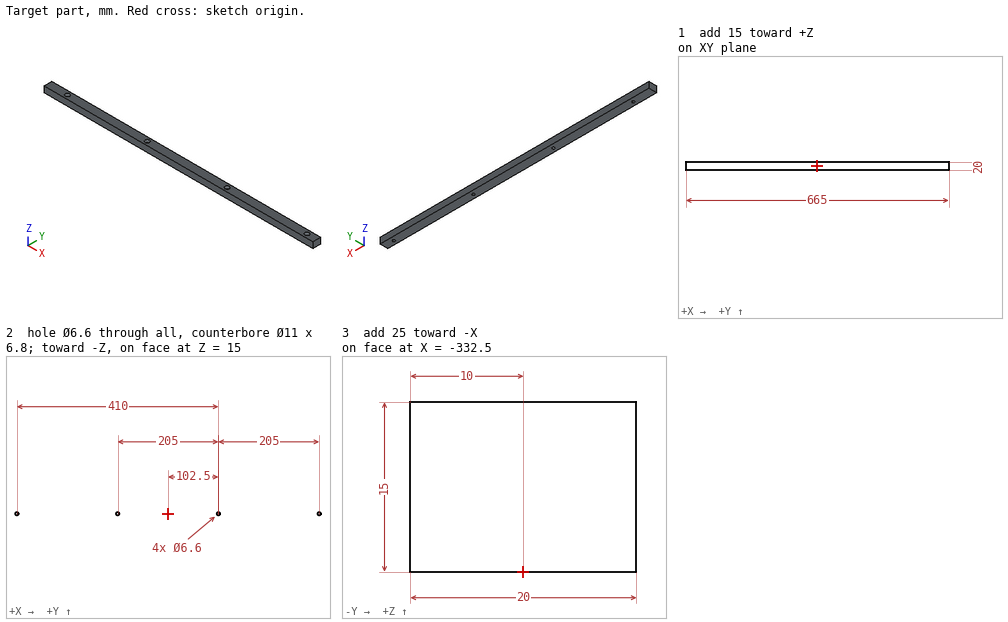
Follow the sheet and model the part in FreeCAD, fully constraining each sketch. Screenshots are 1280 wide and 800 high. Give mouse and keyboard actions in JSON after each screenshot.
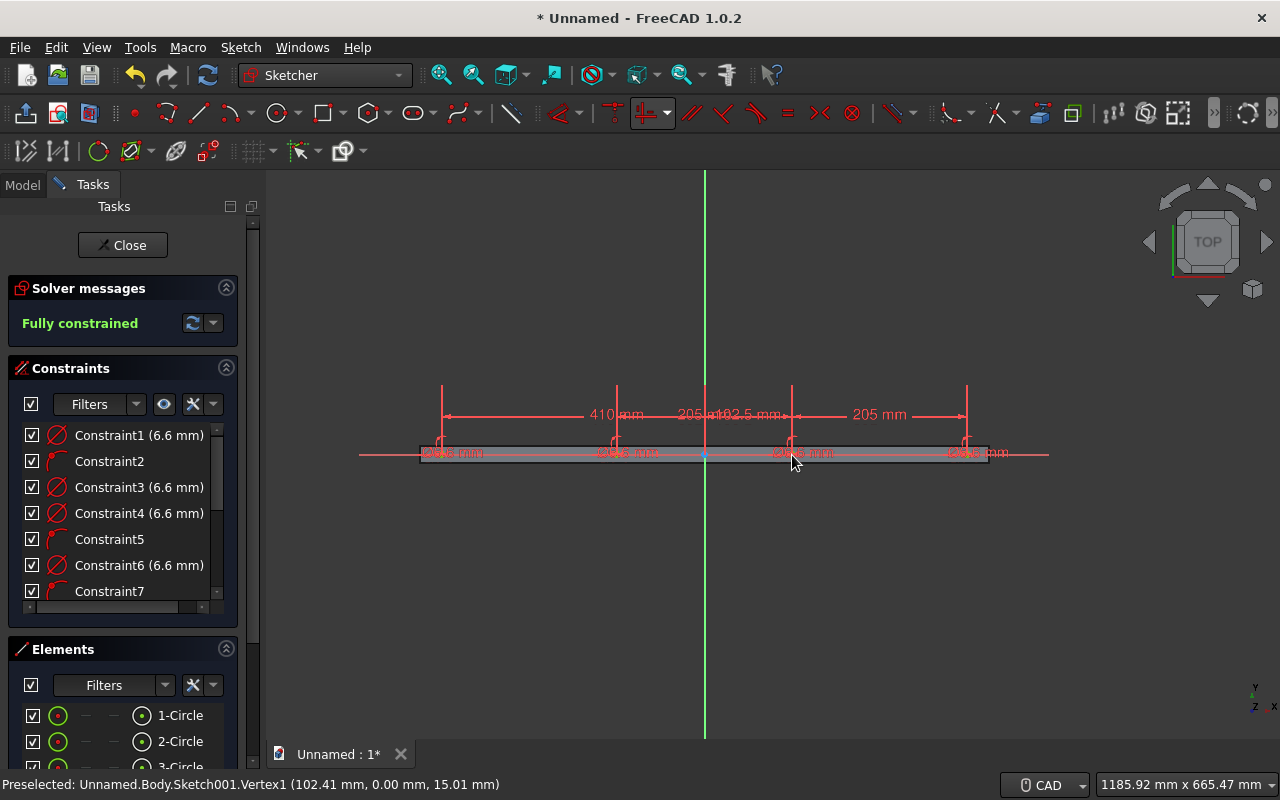
{"action": "left_click", "coordinate": [123, 245]}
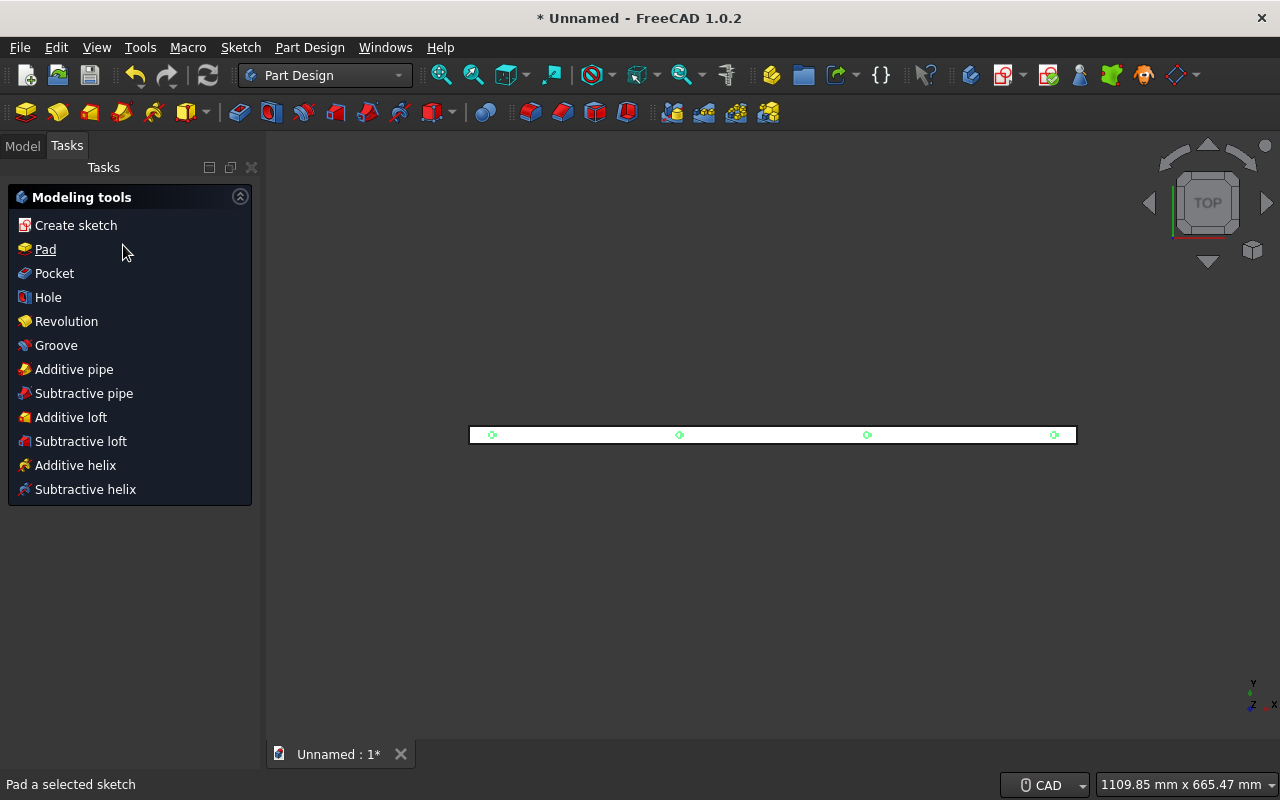
{"action": "left_click", "coordinate": [272, 112]}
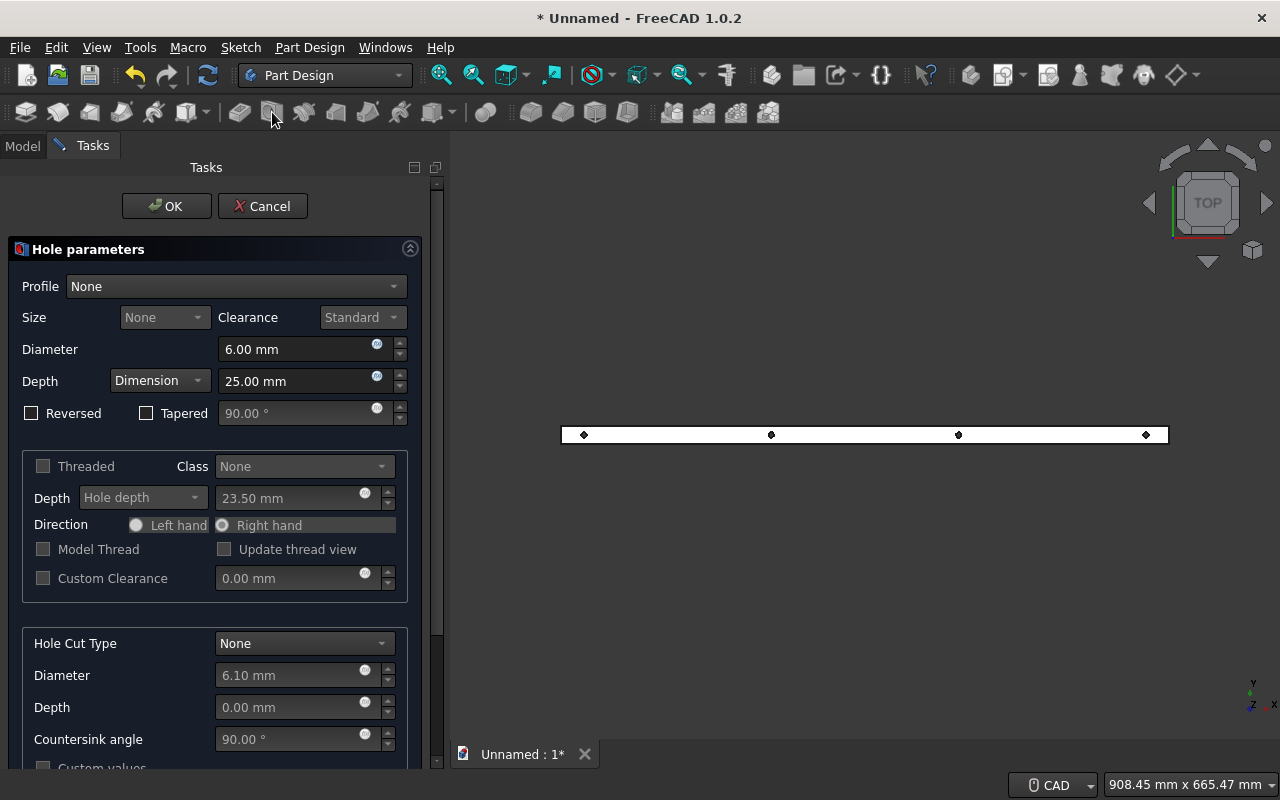
{"action": "triple_click", "coordinate": [305, 349]}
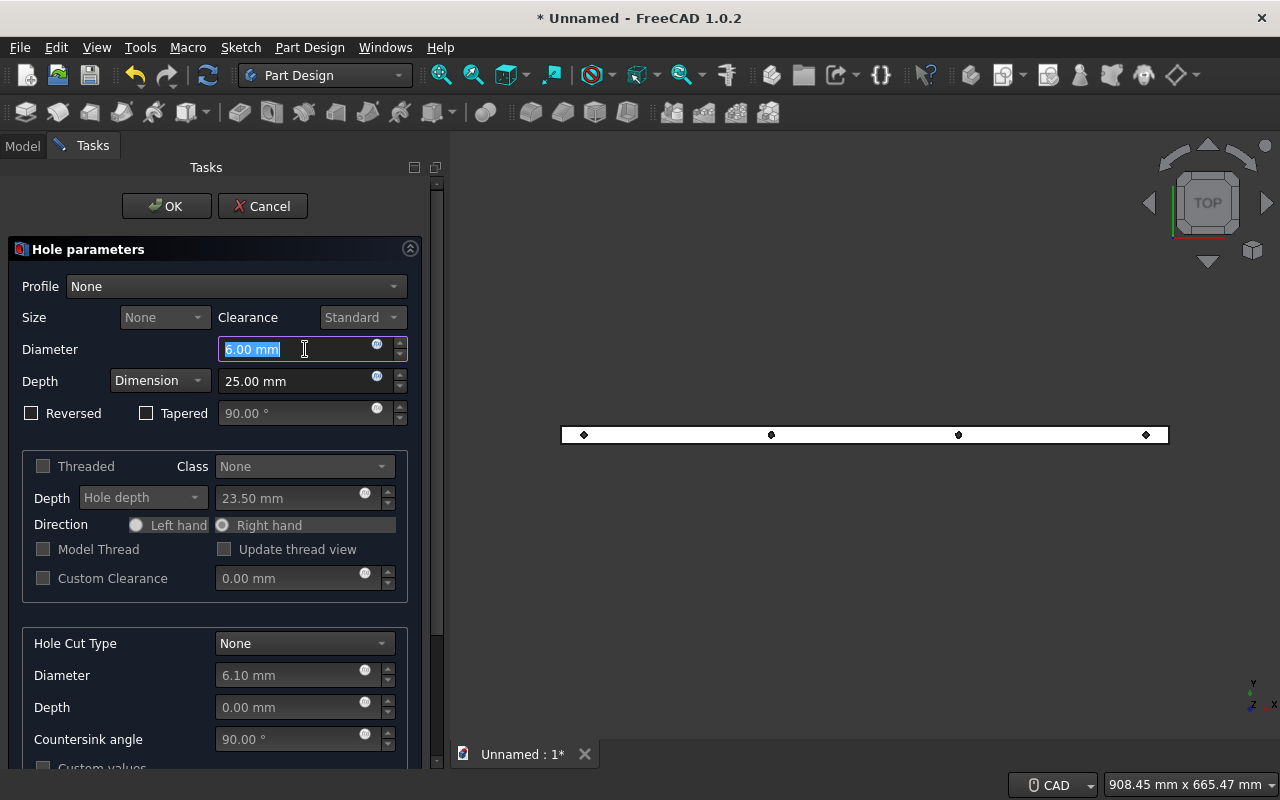
{"action": "type", "text": "6.6"}
{"action": "key", "text": "Tab"}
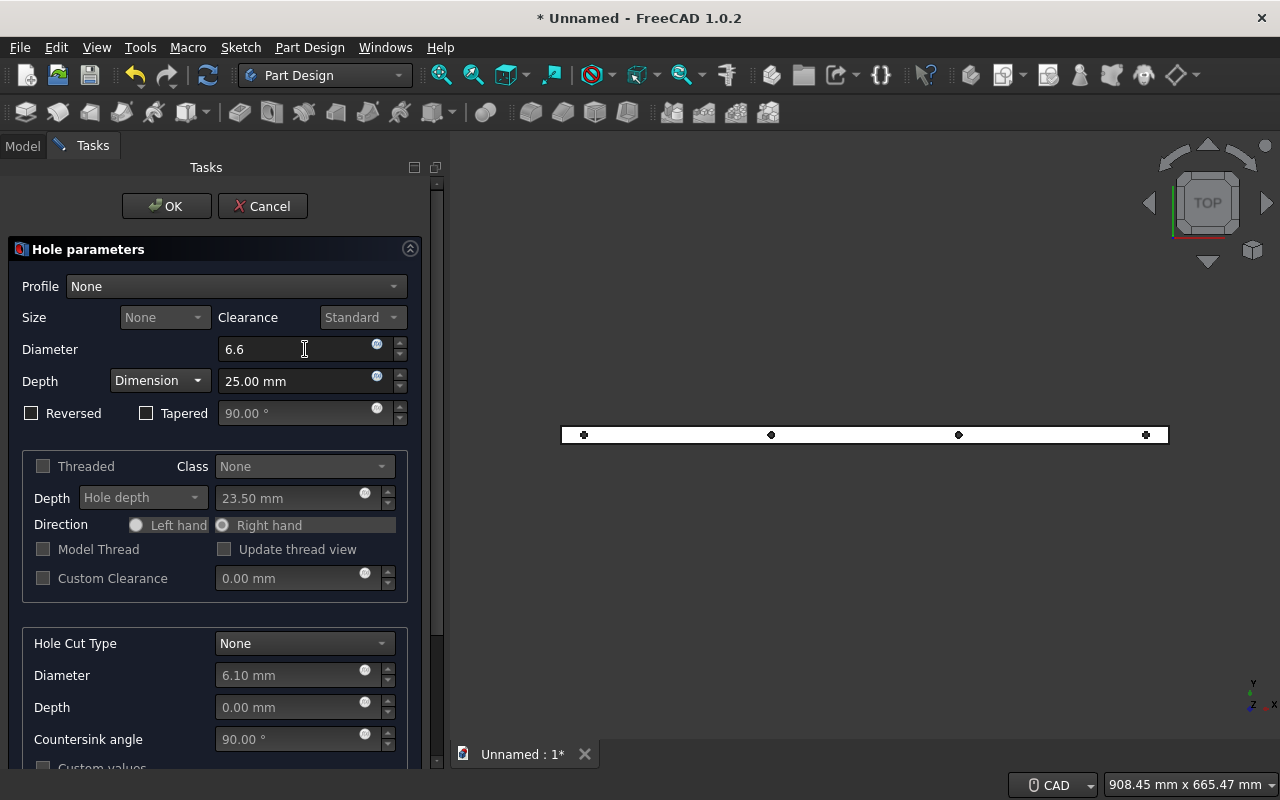
{"action": "left_click", "coordinate": [161, 380]}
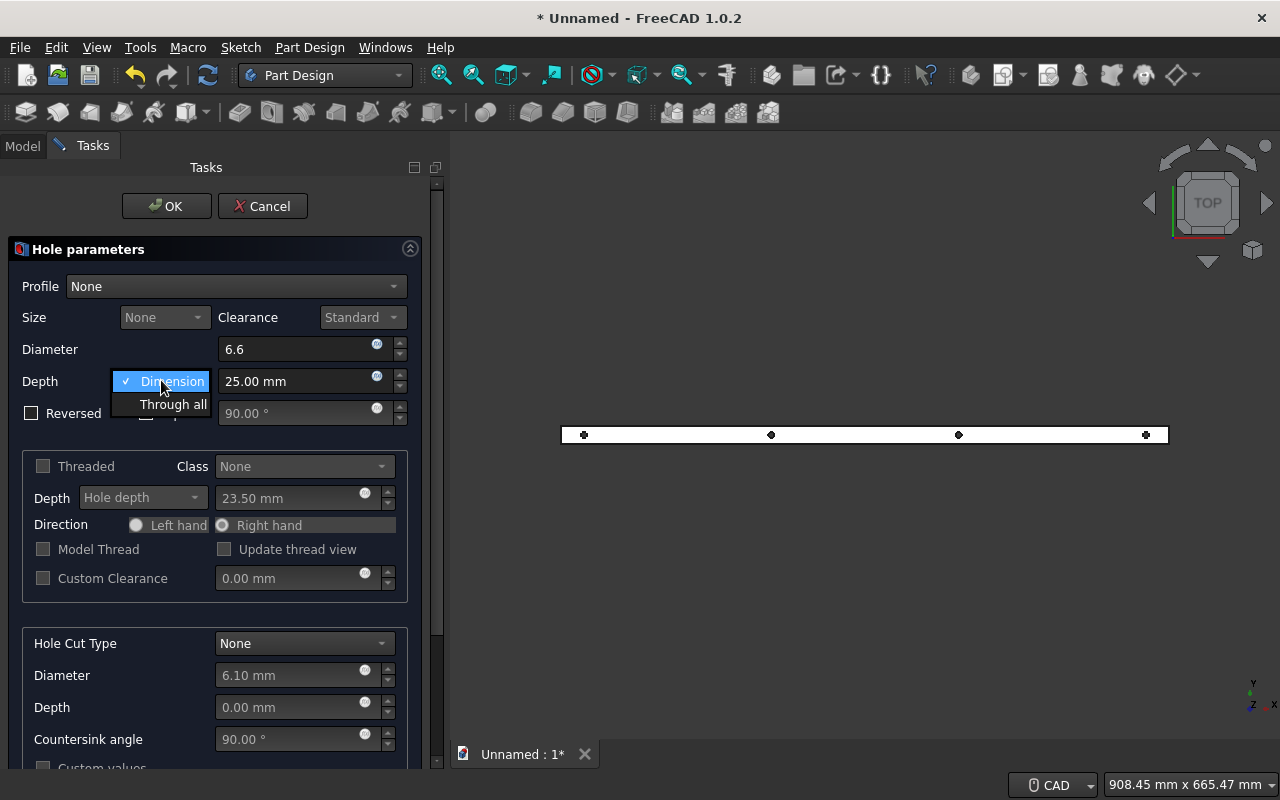
{"action": "left_click", "coordinate": [160, 404]}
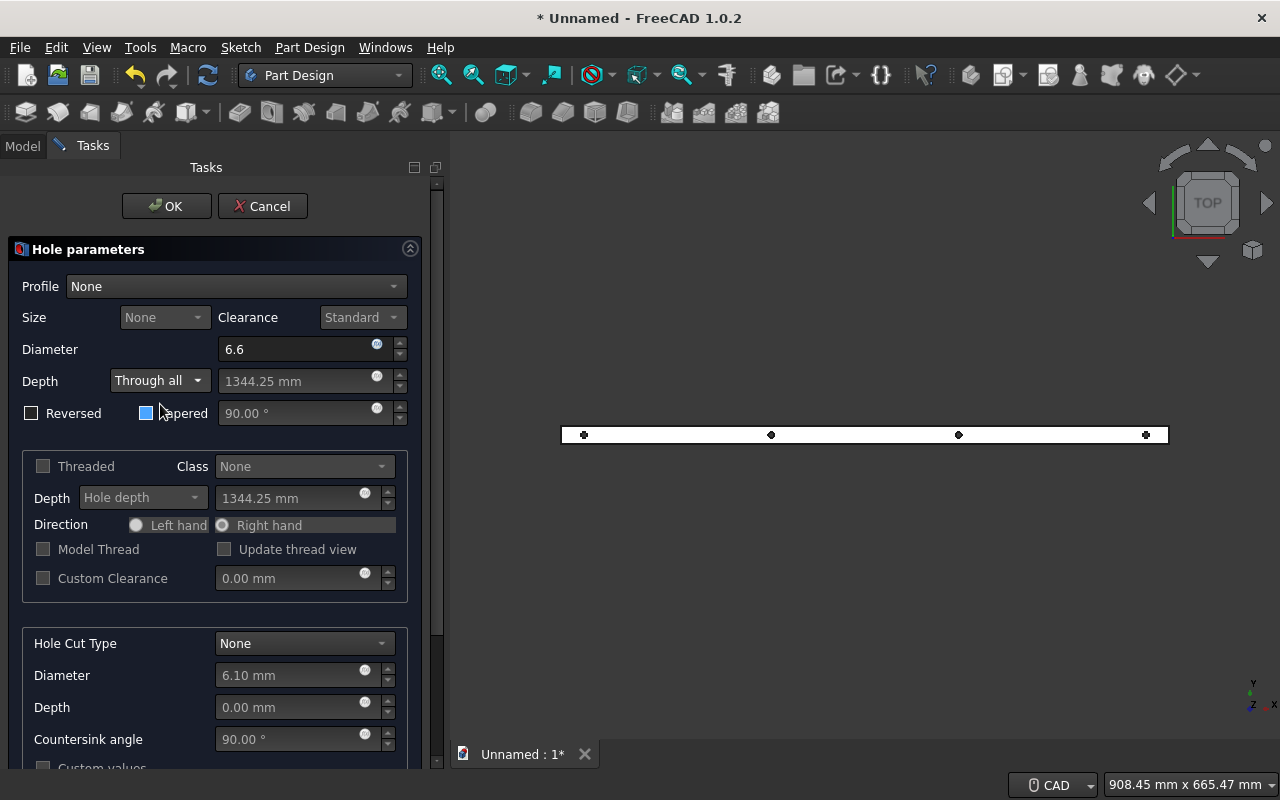
{"action": "left_click", "coordinate": [306, 644]}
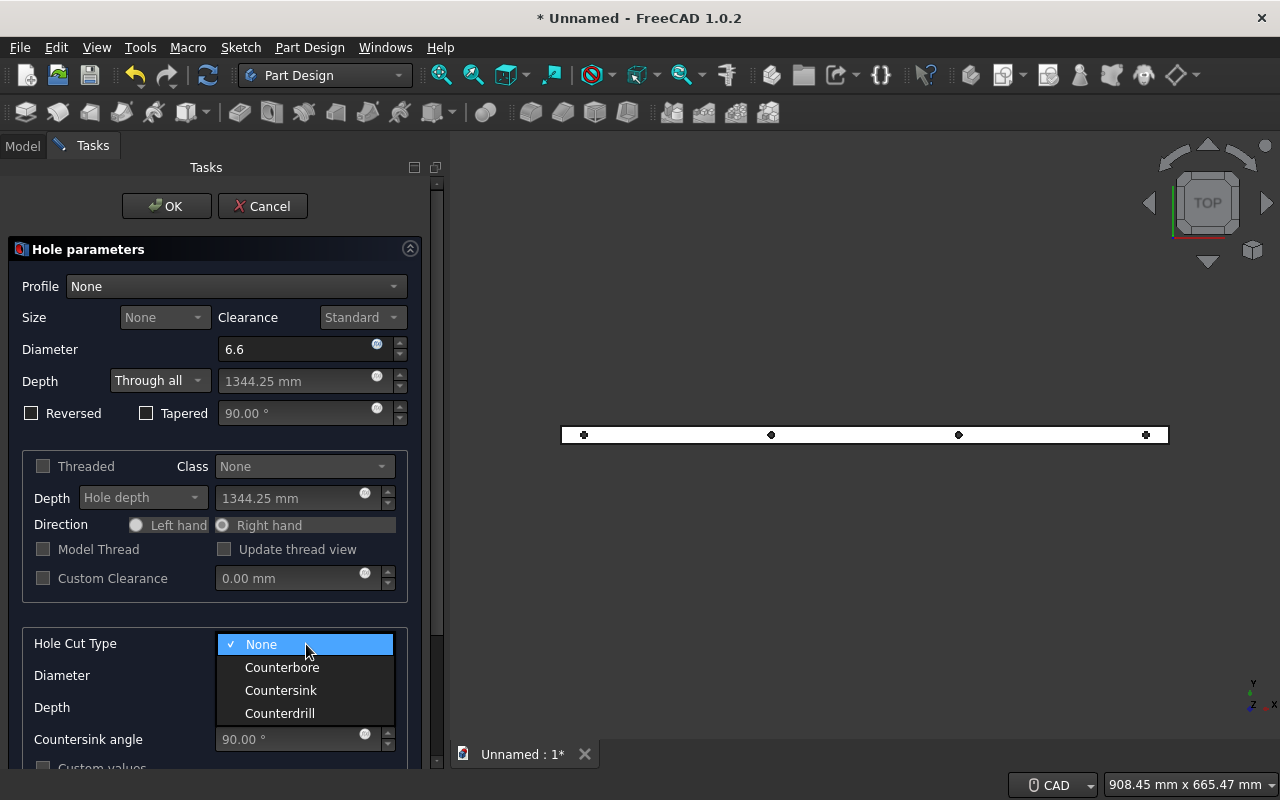
{"action": "left_click", "coordinate": [304, 668]}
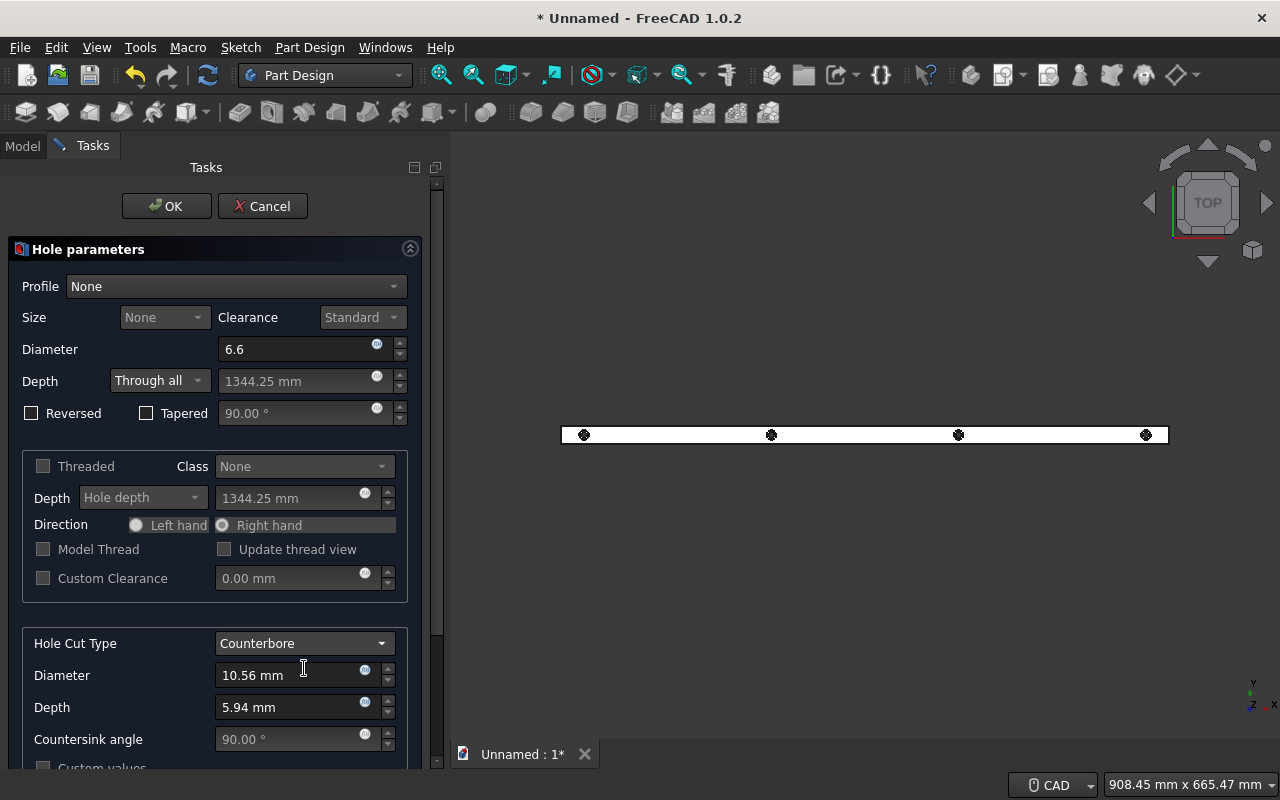
{"action": "triple_click", "coordinate": [298, 675]}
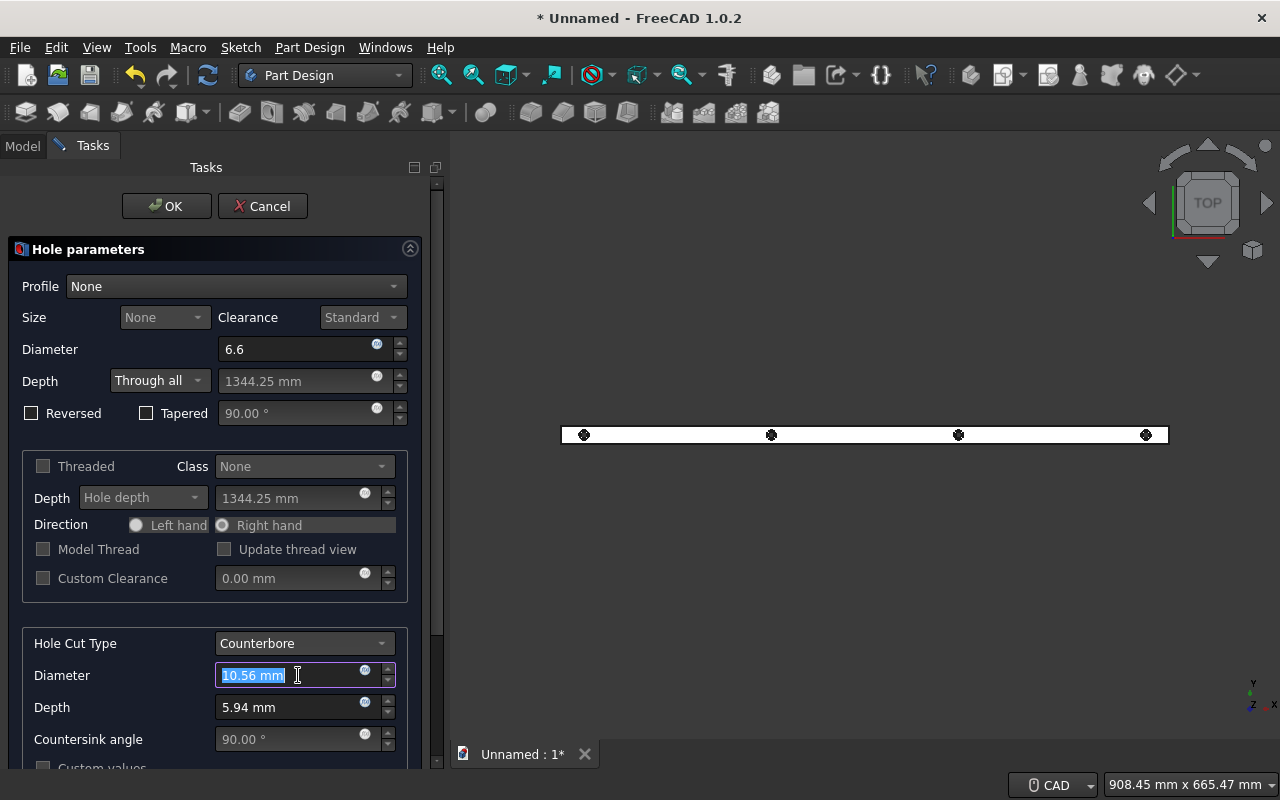
{"action": "type", "text": "11"}
{"action": "key", "text": "Tab"}